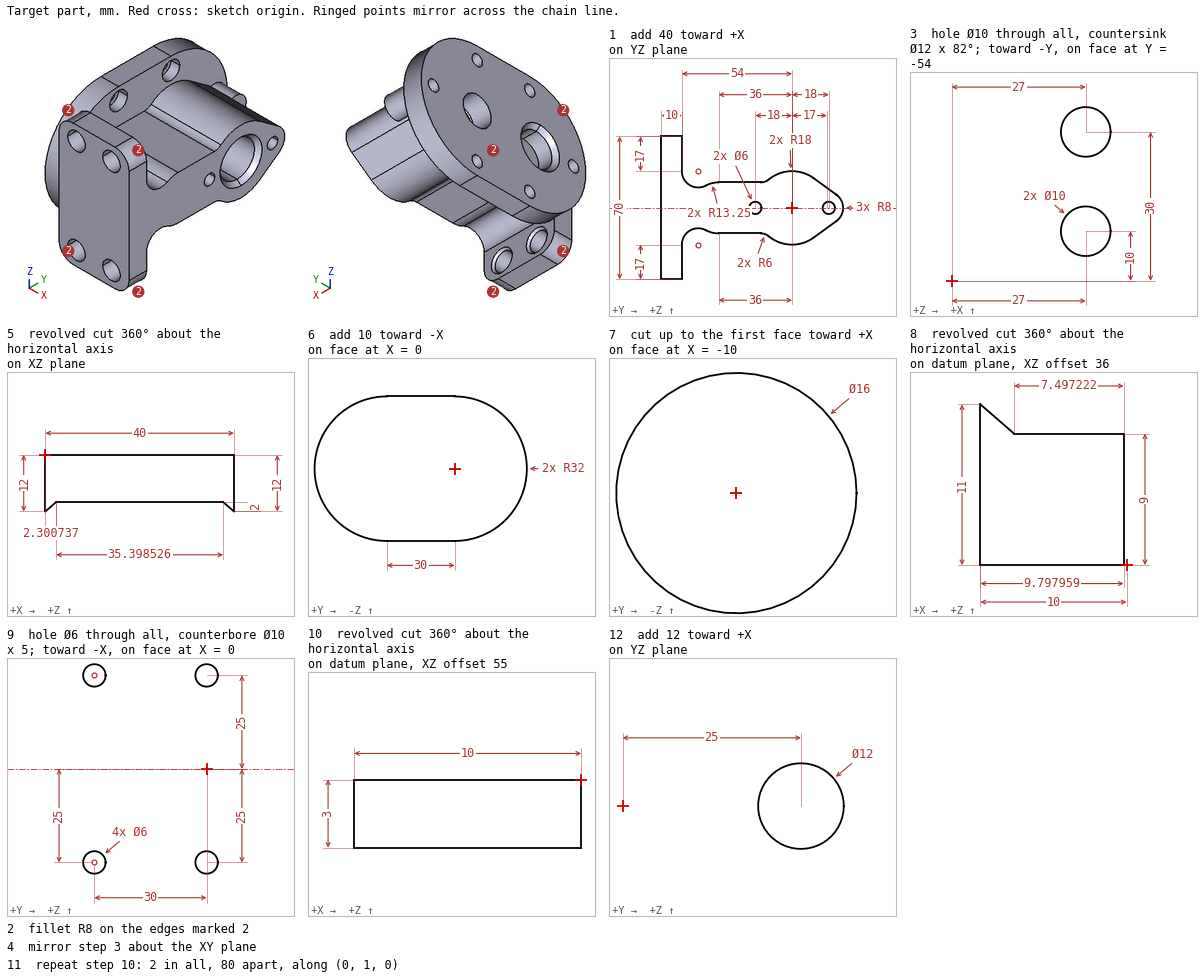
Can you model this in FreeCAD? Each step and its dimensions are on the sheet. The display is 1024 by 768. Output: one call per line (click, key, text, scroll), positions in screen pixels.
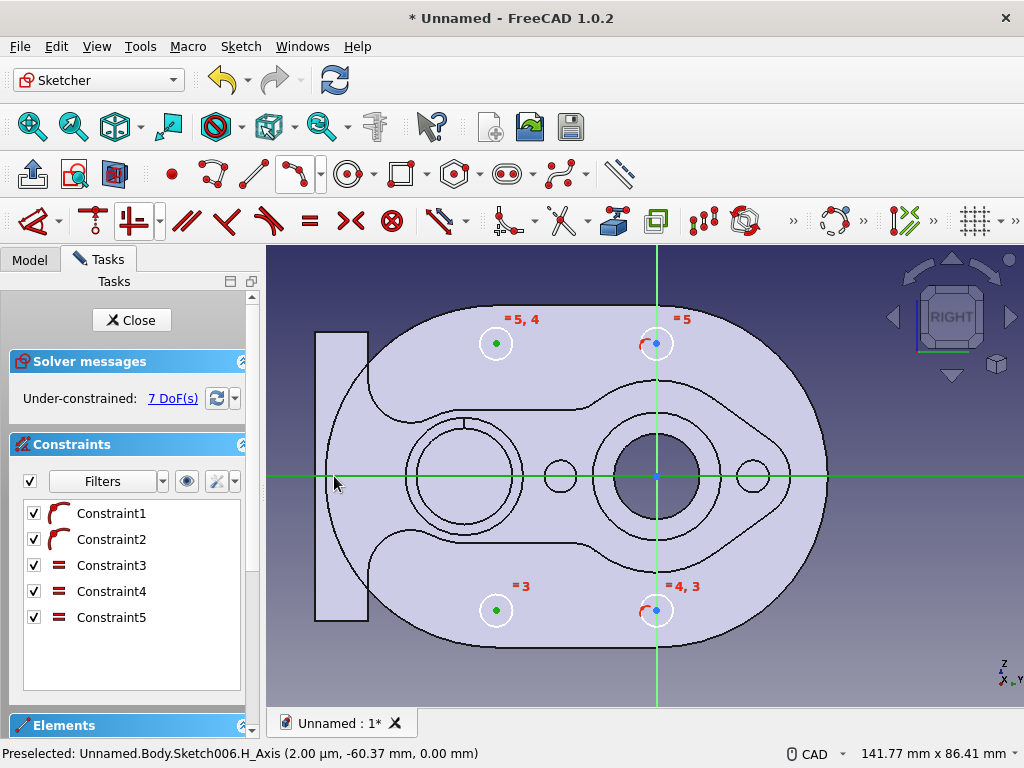
click(351, 222)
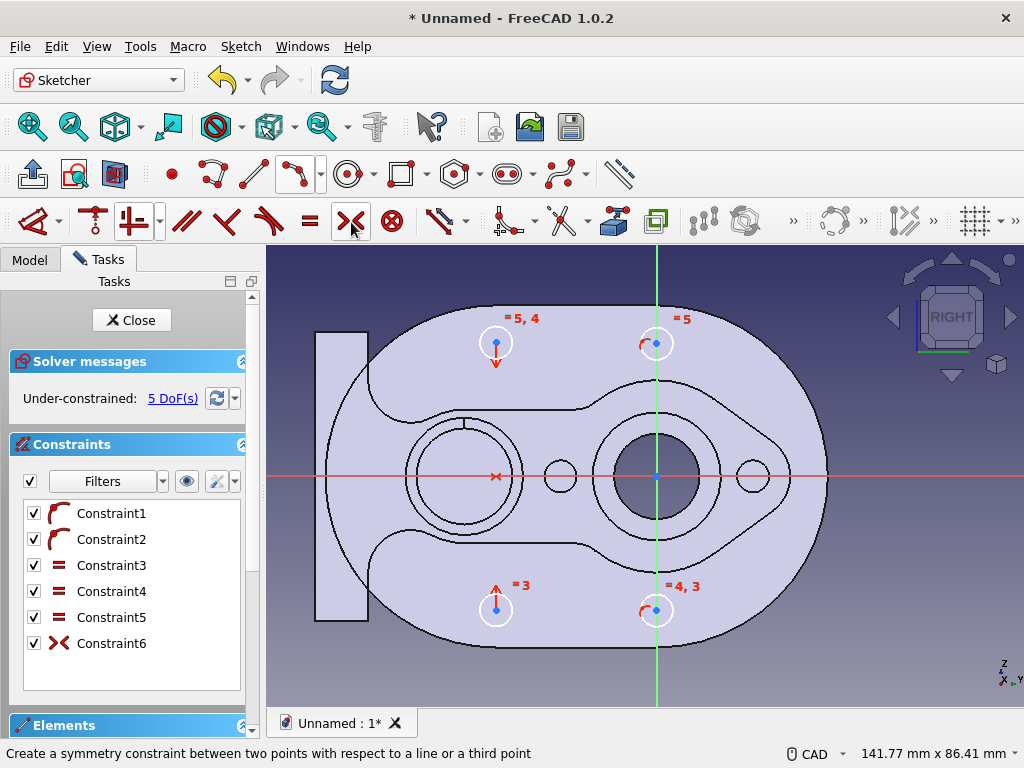
click(32, 222)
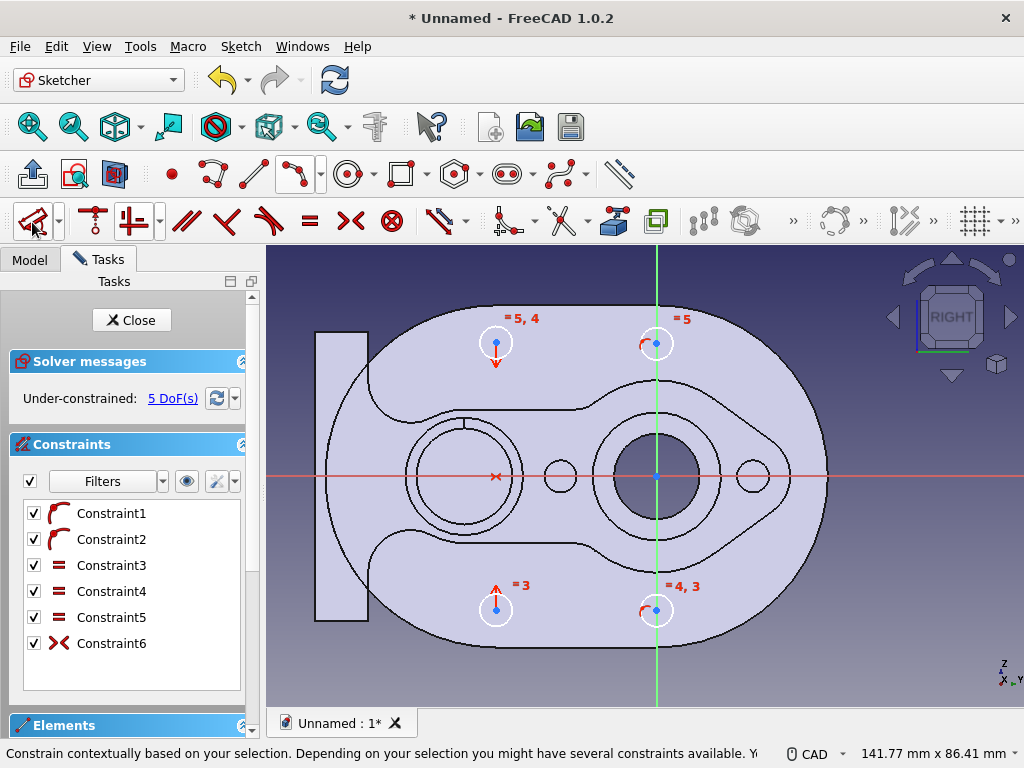
scroll(507, 599, up, 2)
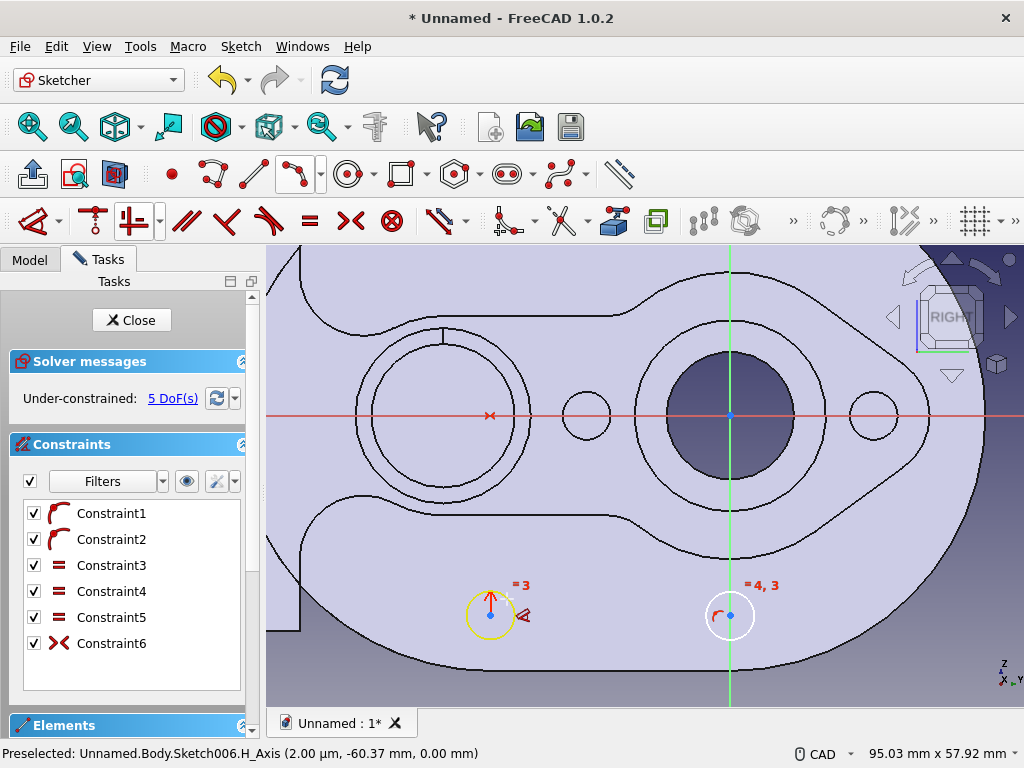
click(508, 598)
click(531, 575)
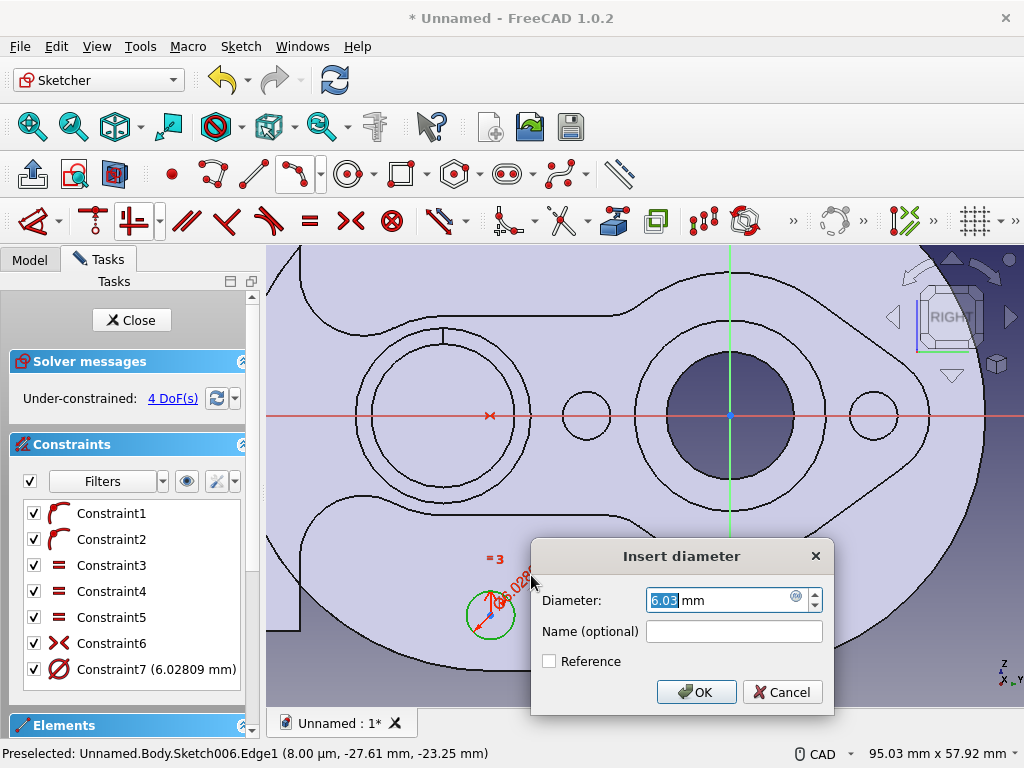
text(6)
key(Return)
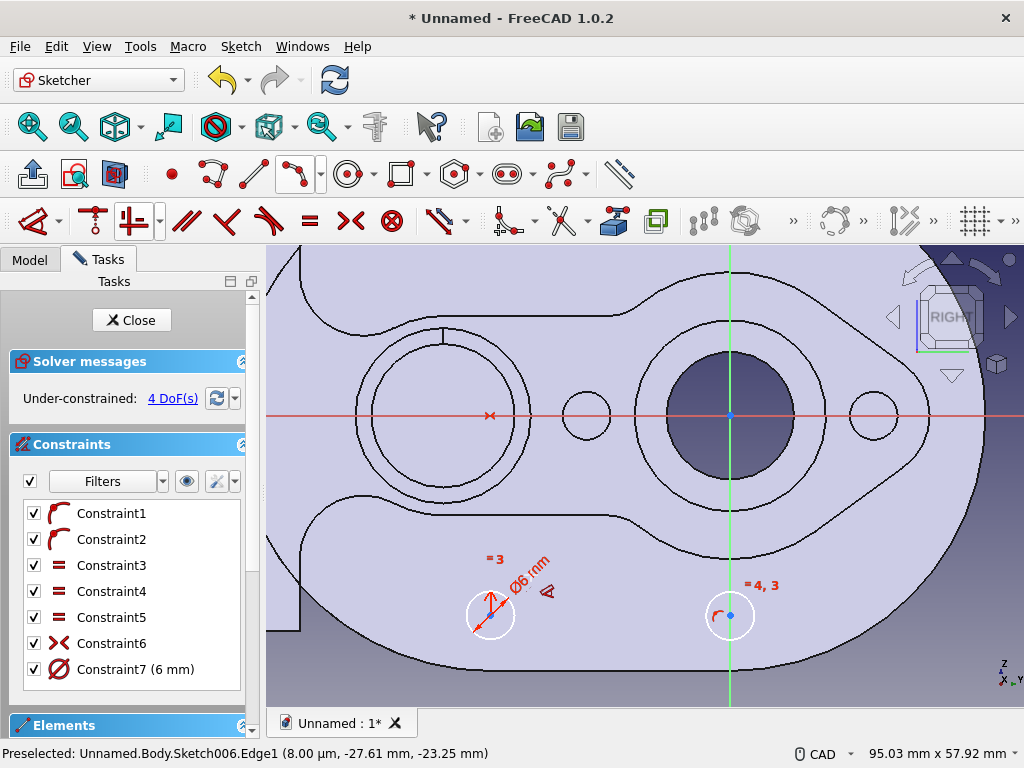
click(491, 615)
click(610, 649)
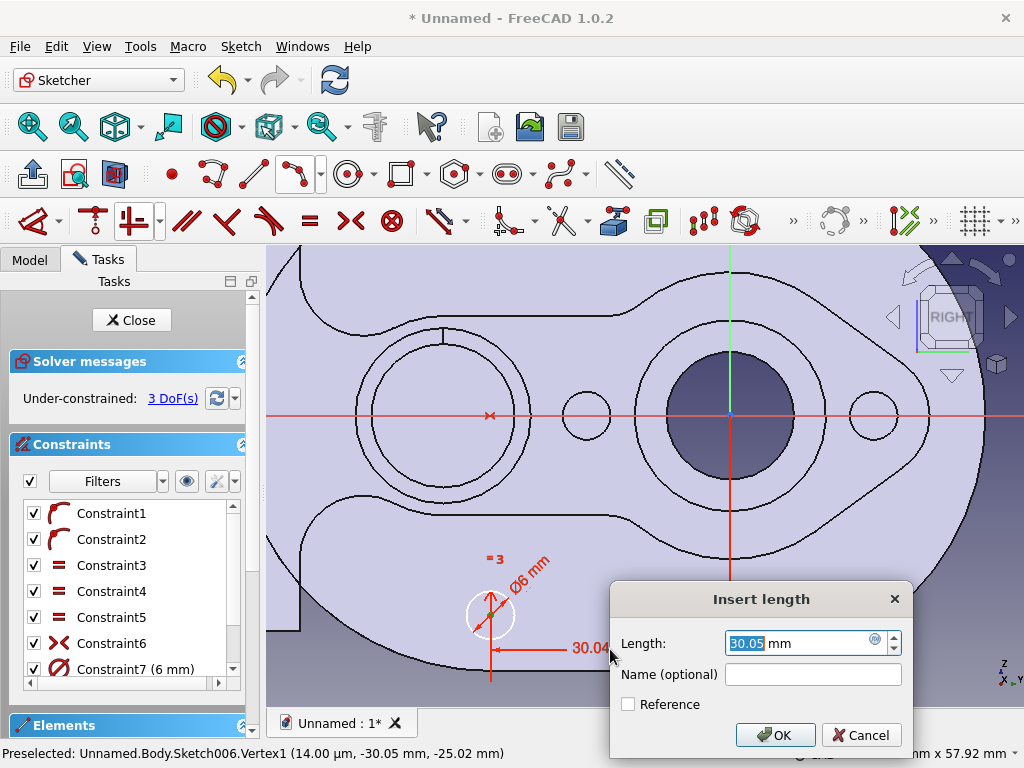
text(30)
key(Return)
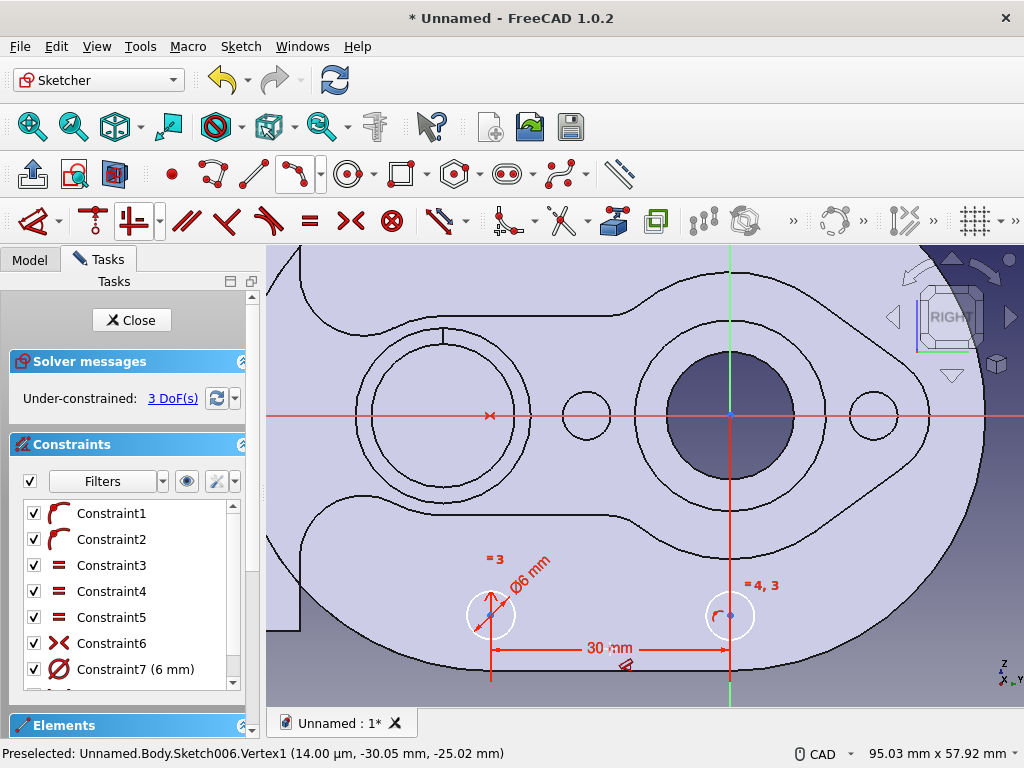
click(491, 615)
click(764, 516)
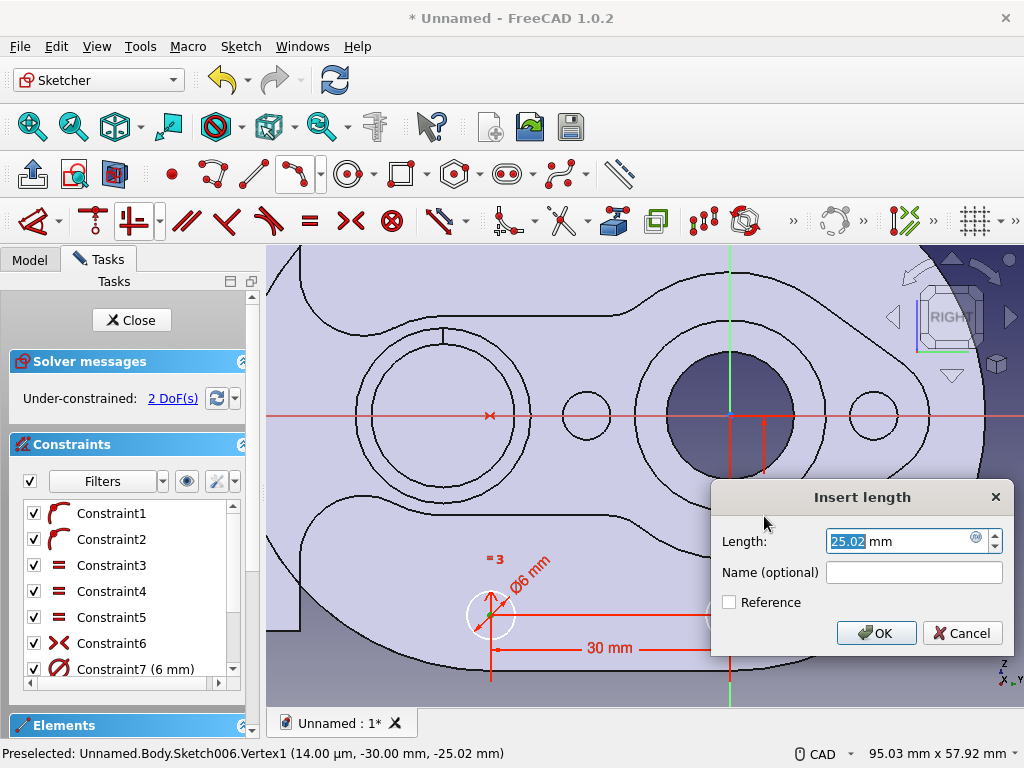
text(25)
key(Return)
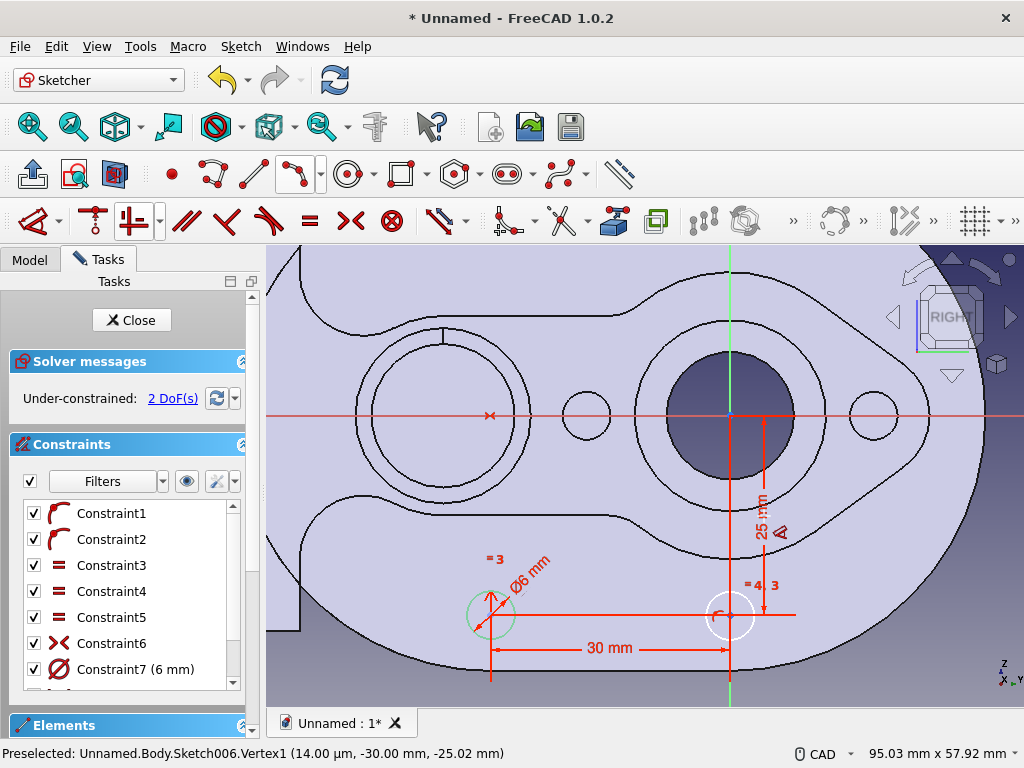
click(730, 616)
click(764, 470)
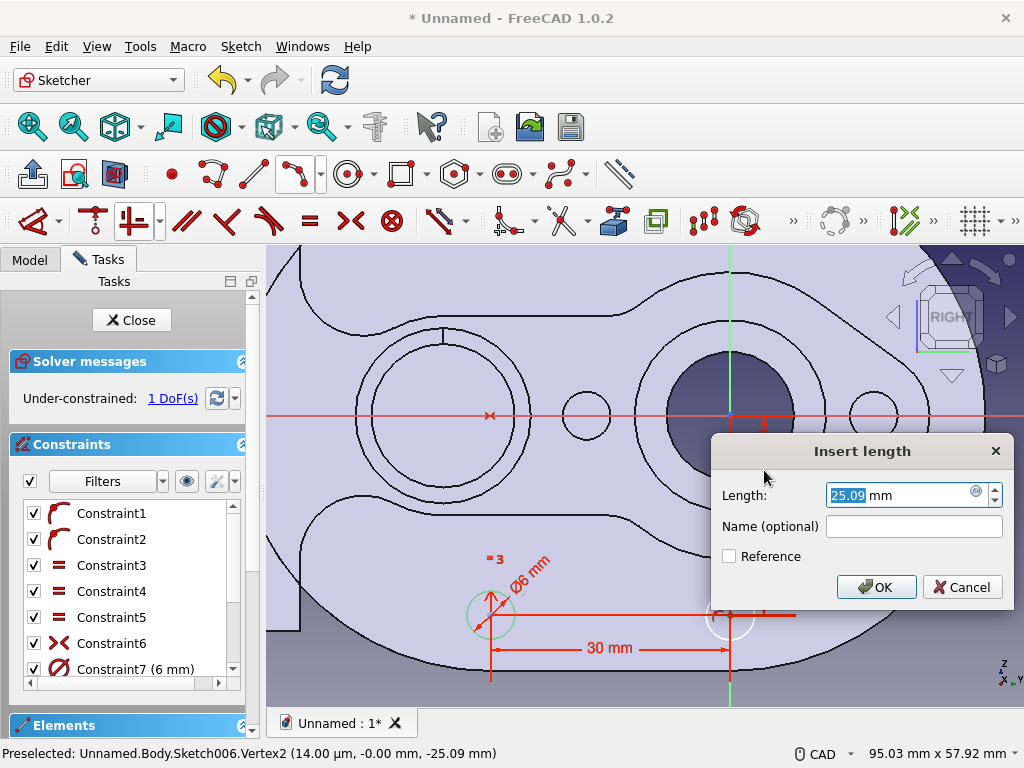
text(25)
key(Return)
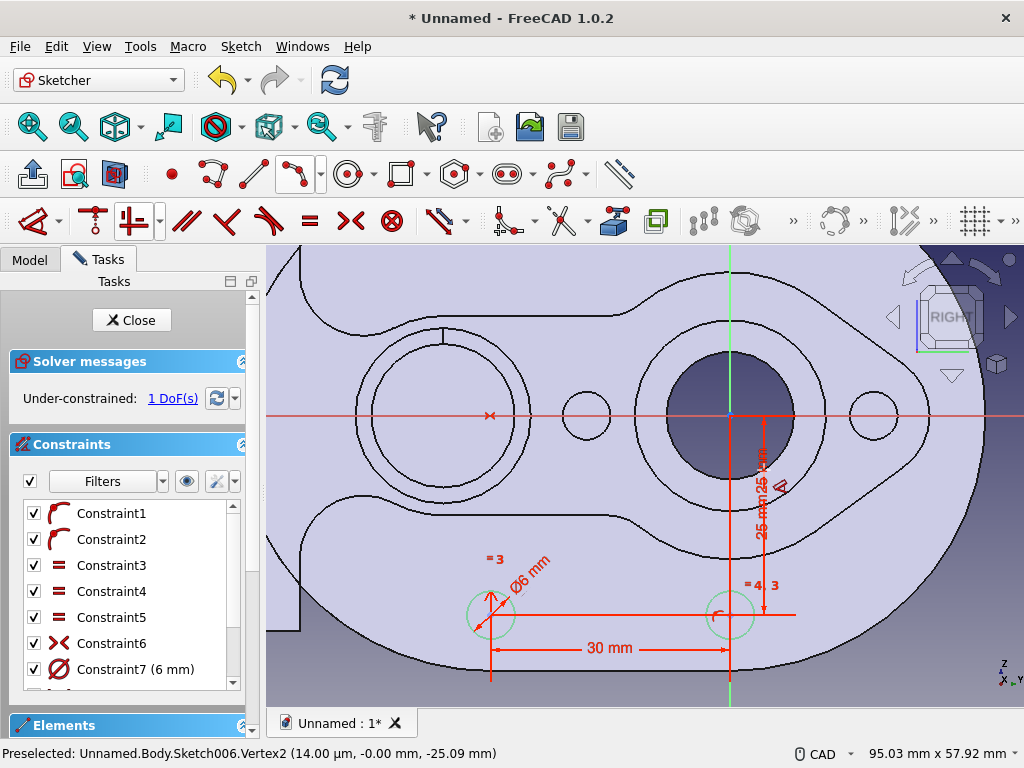
scroll(507, 599, down, 2)